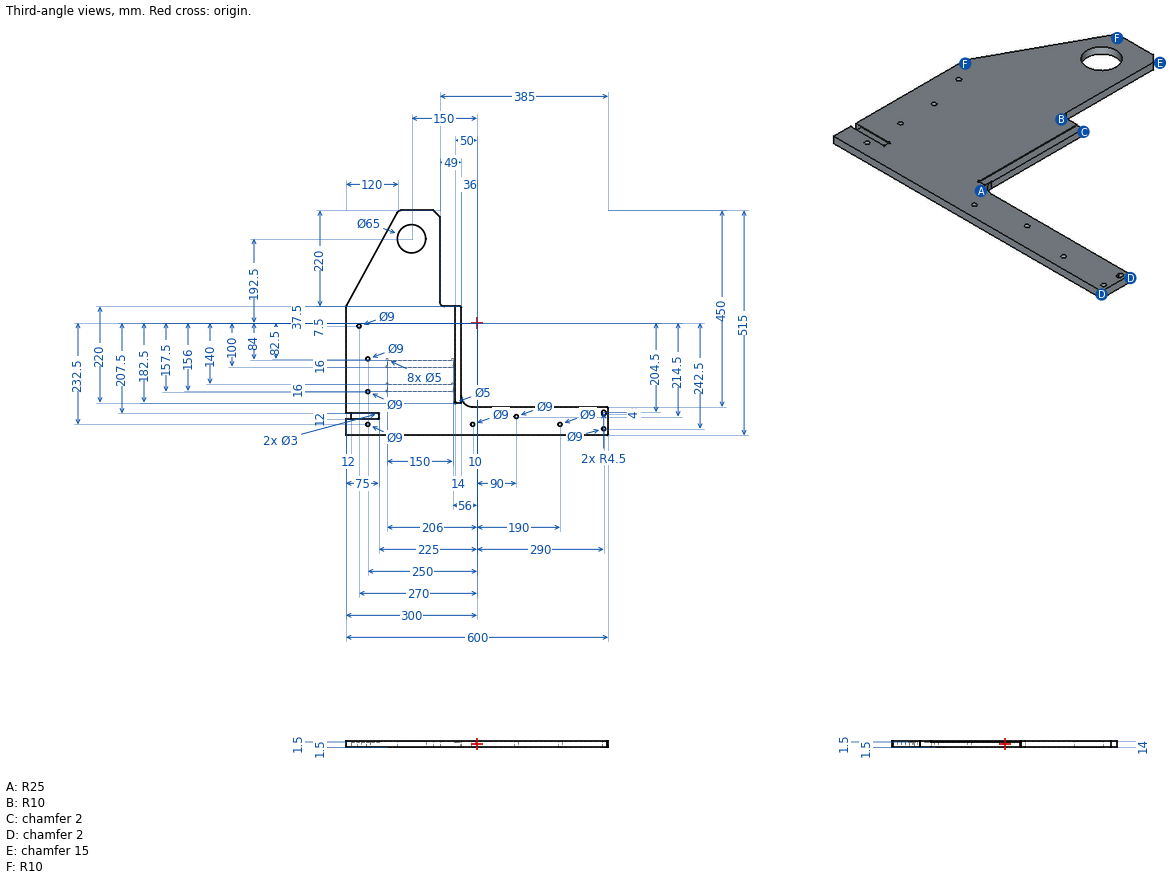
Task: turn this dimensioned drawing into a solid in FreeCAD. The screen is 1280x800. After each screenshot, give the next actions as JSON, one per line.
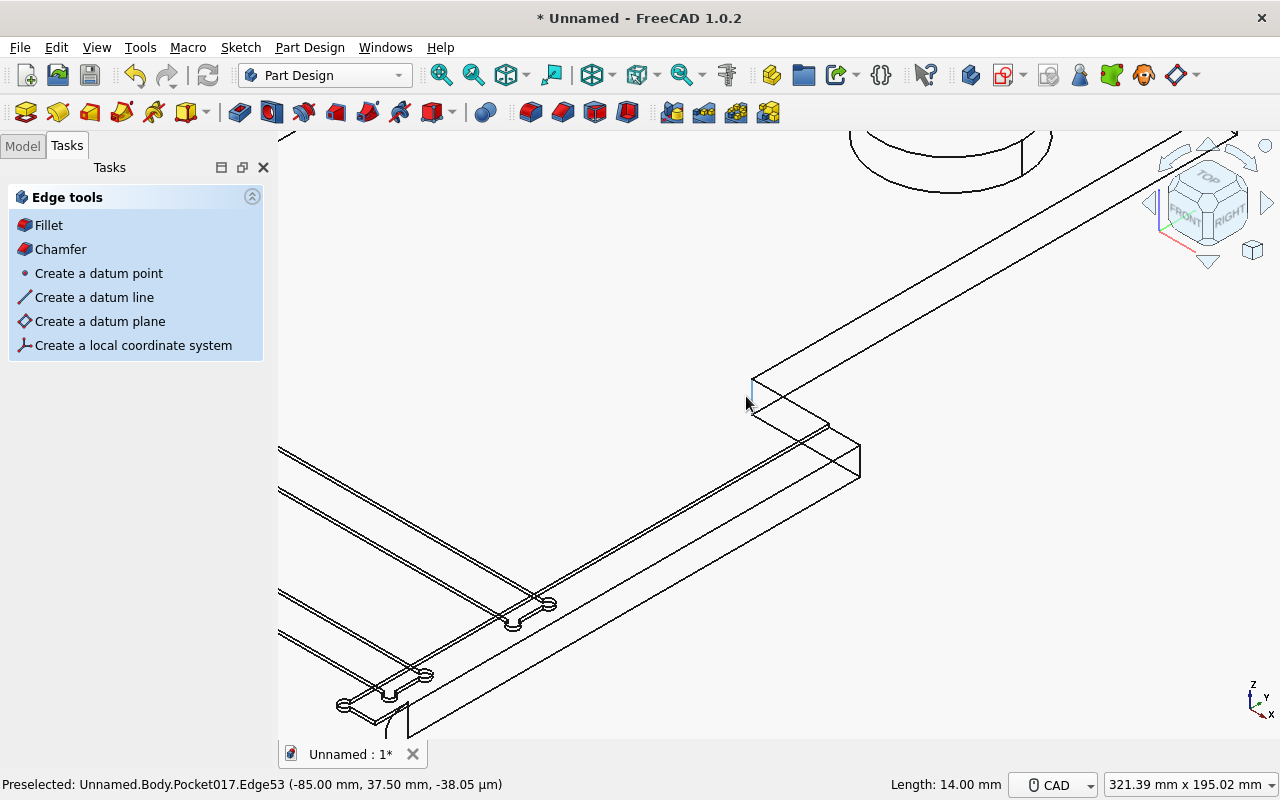
{"action": "key", "text": "v 1"}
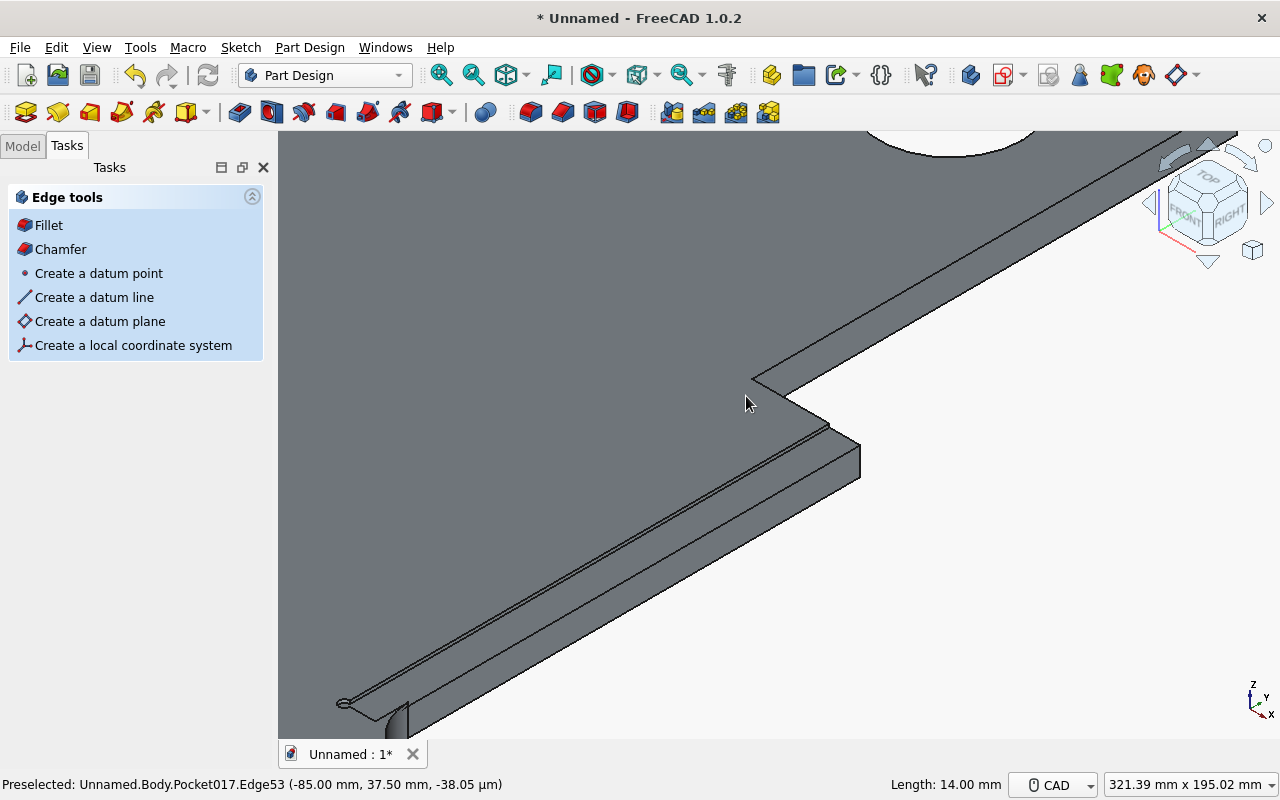
{"action": "left_click", "coordinate": [532, 112]}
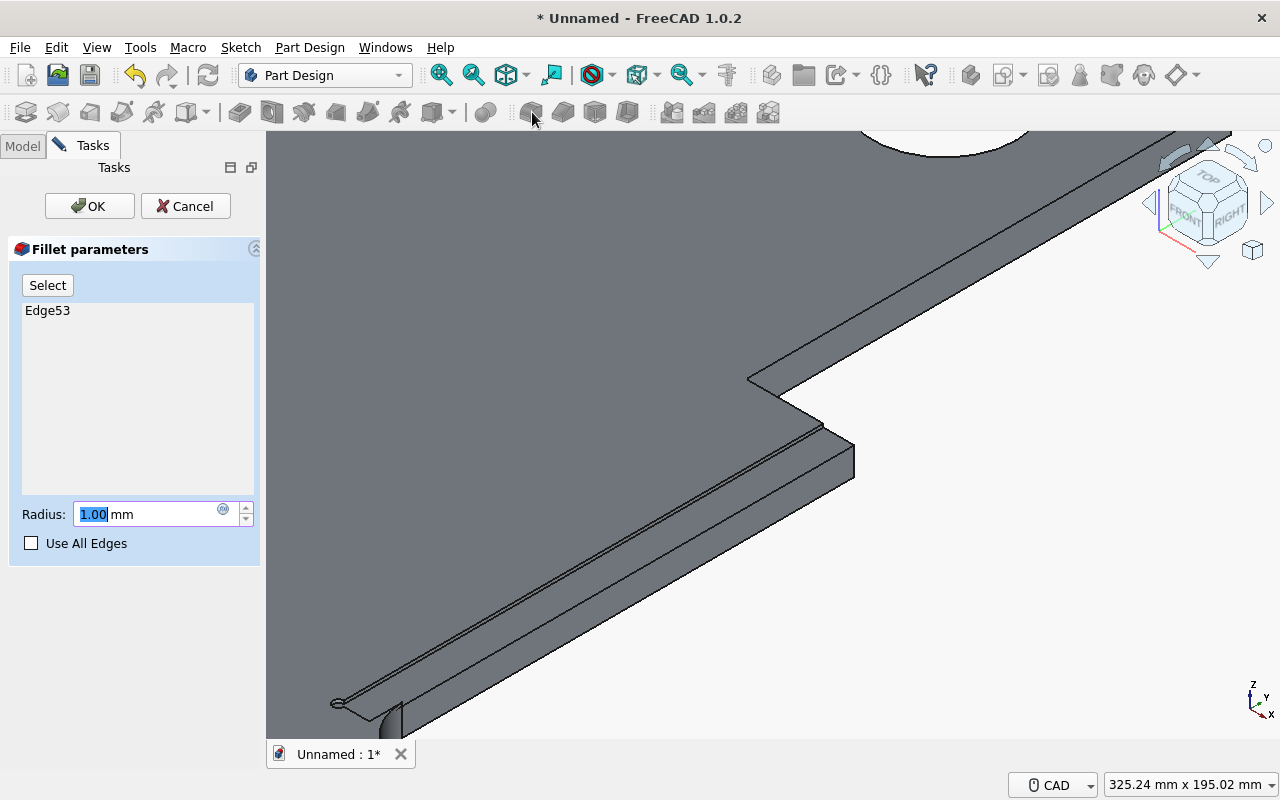
{"action": "type", "text": "10"}
{"action": "key", "text": "Tab"}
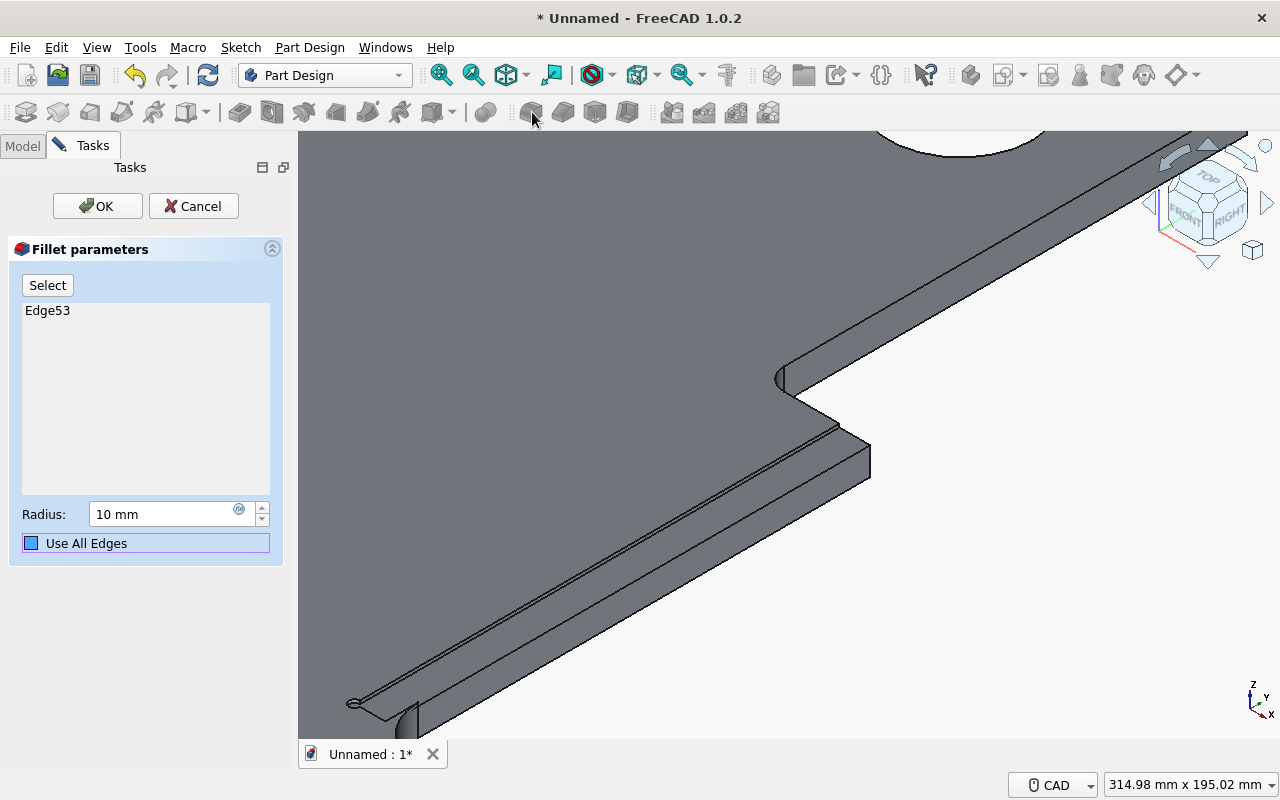
{"action": "left_click", "coordinate": [98, 206]}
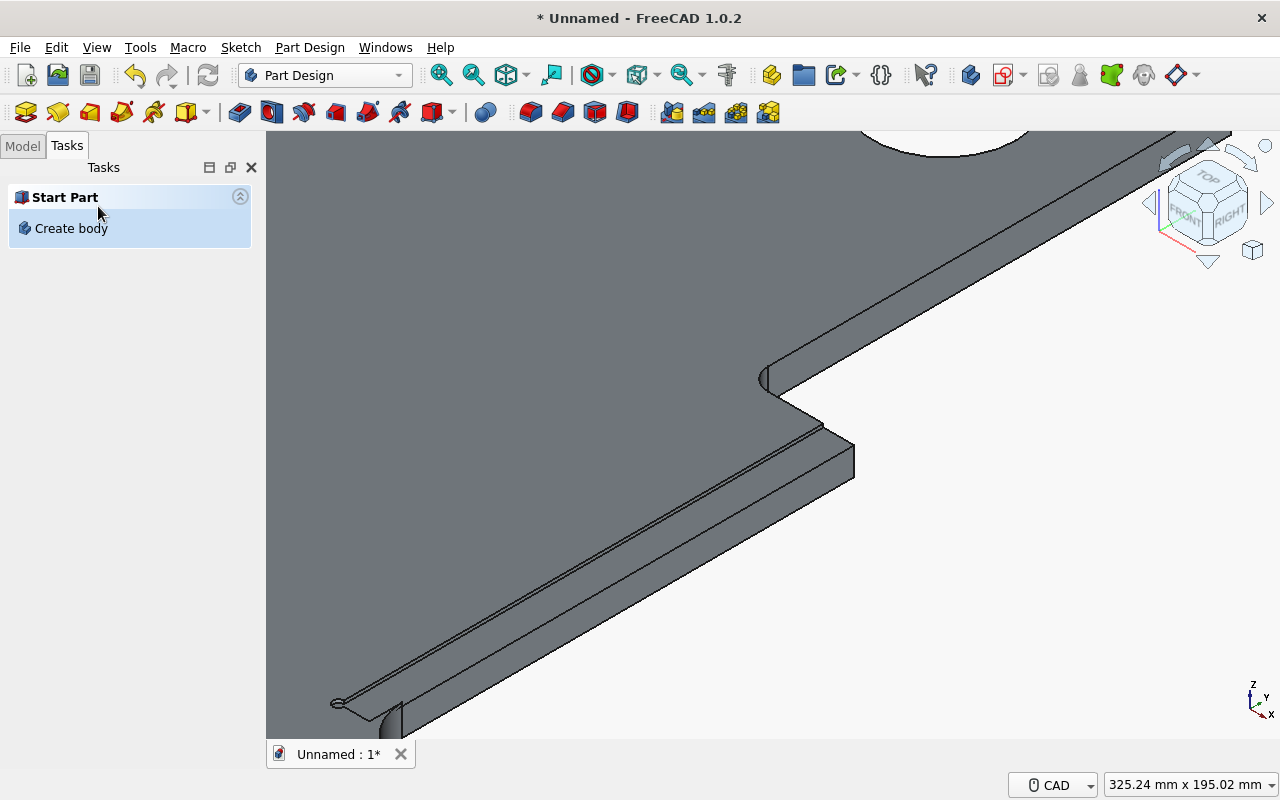
{"action": "left_click", "coordinate": [442, 76]}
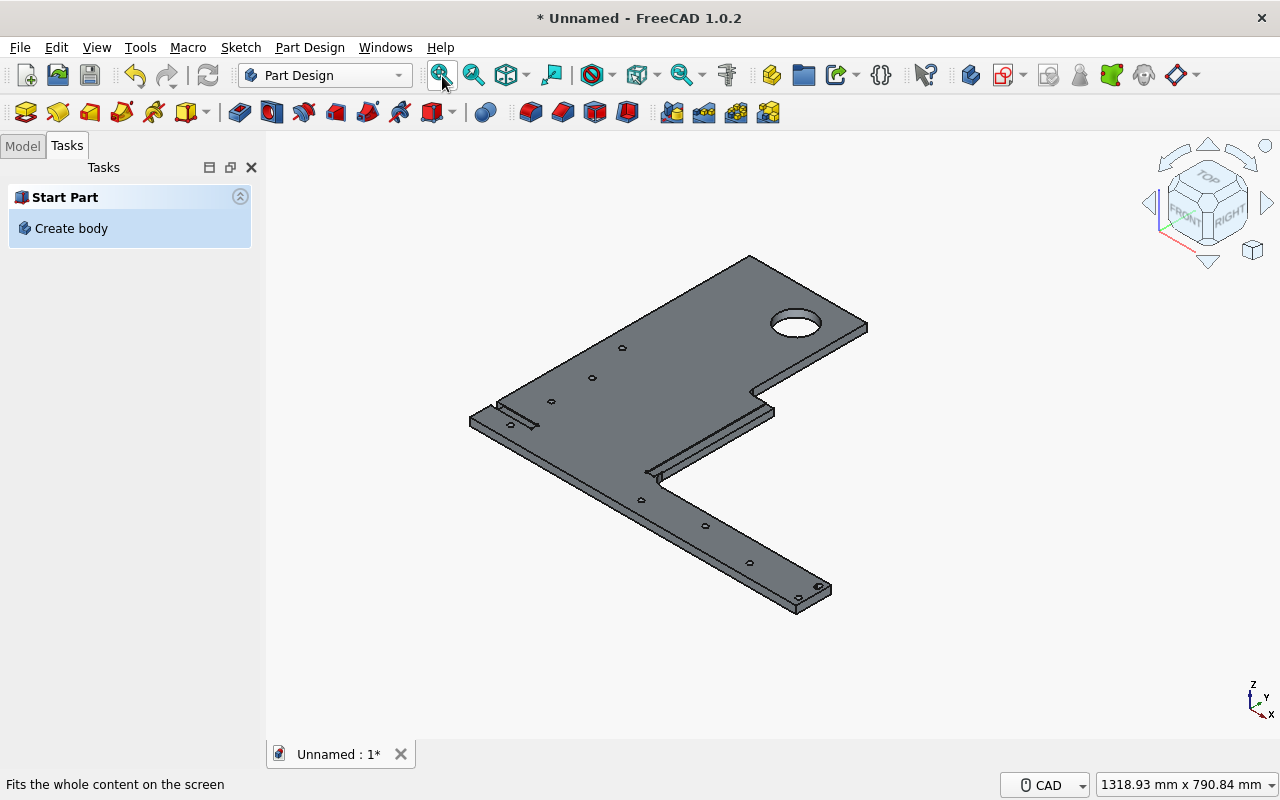
{"action": "scroll", "coordinate": [774, 411], "scroll_direction": "up", "scroll_amount": 8}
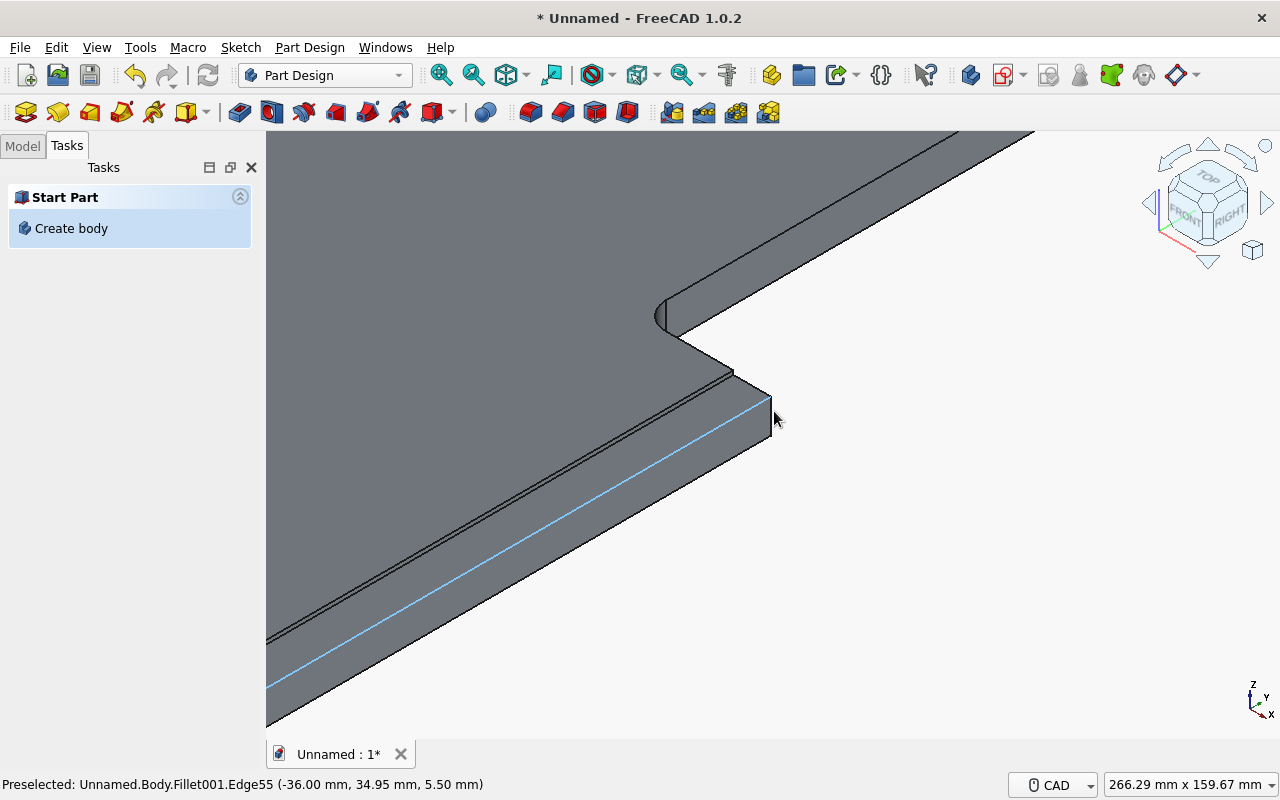
{"action": "left_click", "coordinate": [442, 76]}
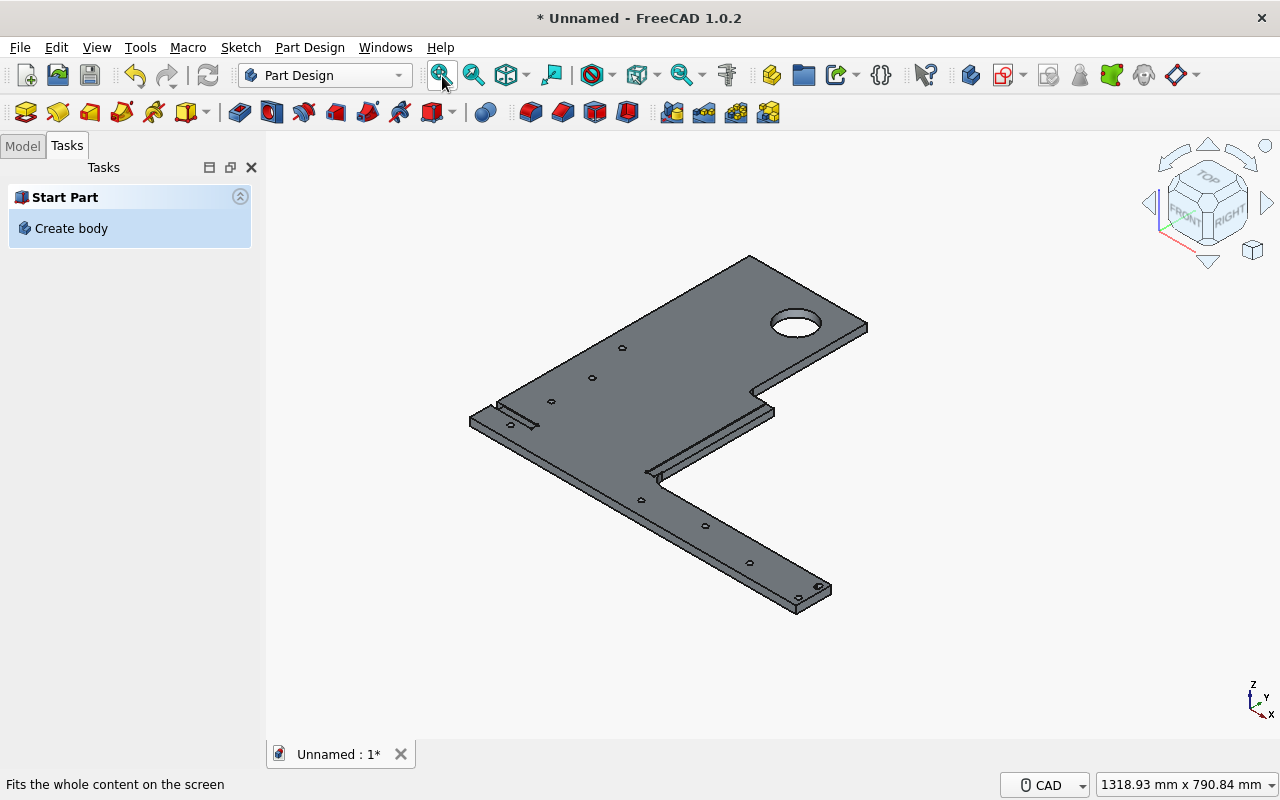
{"action": "key", "text": "2"}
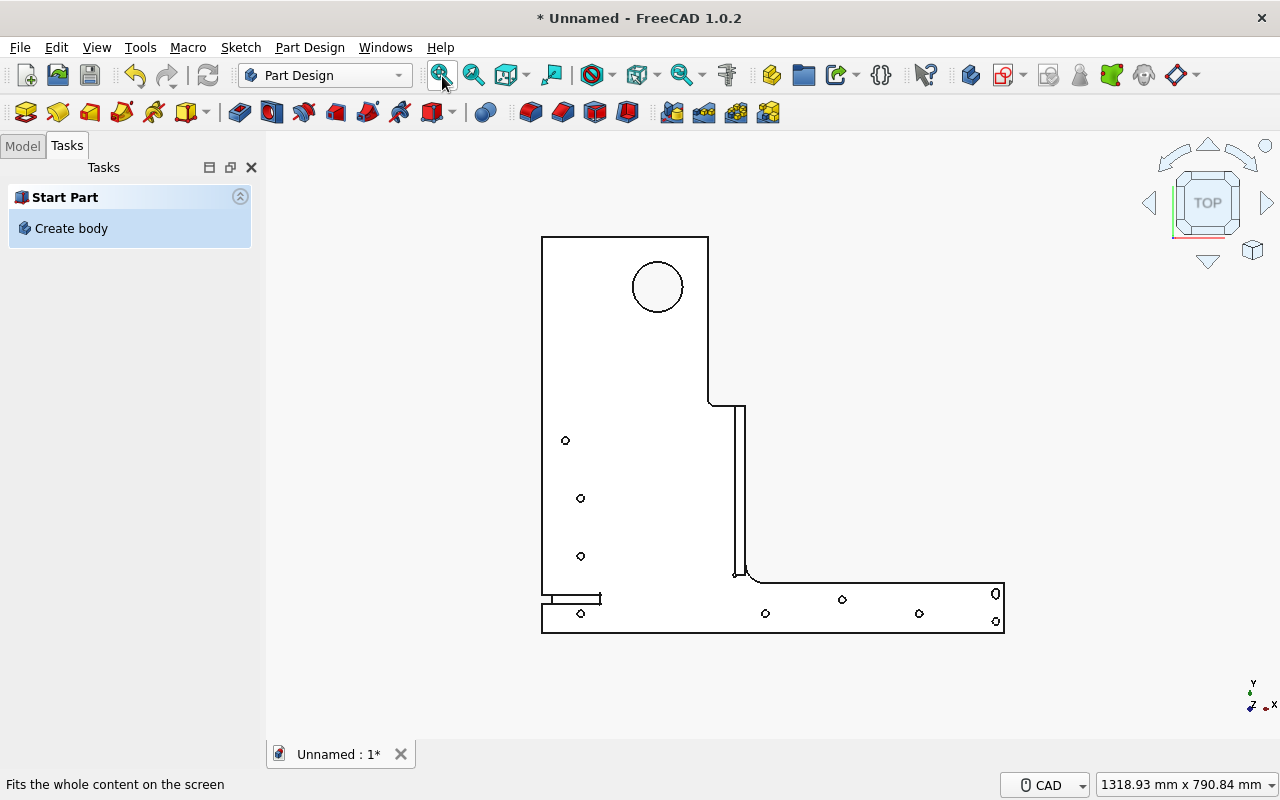
{"action": "scroll", "coordinate": [745, 405], "scroll_direction": "up", "scroll_amount": 8}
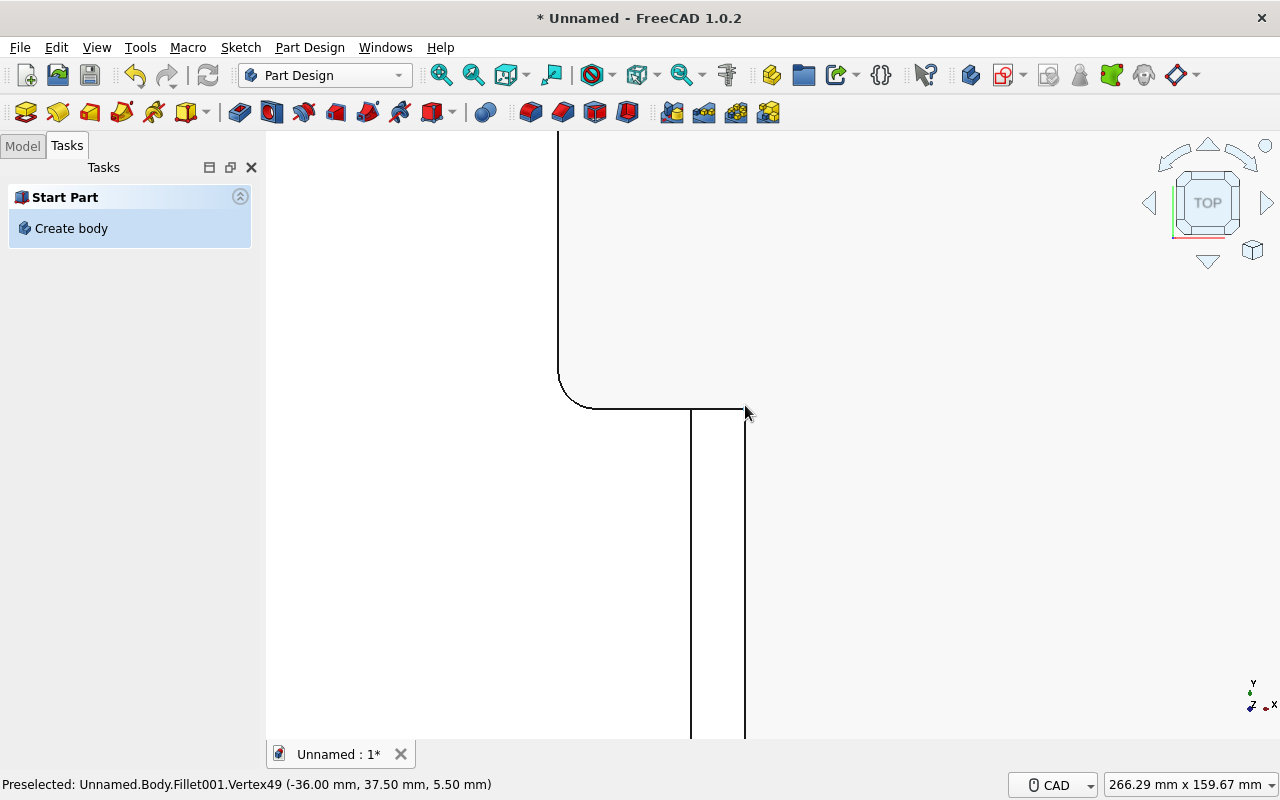
{"action": "left_click", "coordinate": [442, 76]}